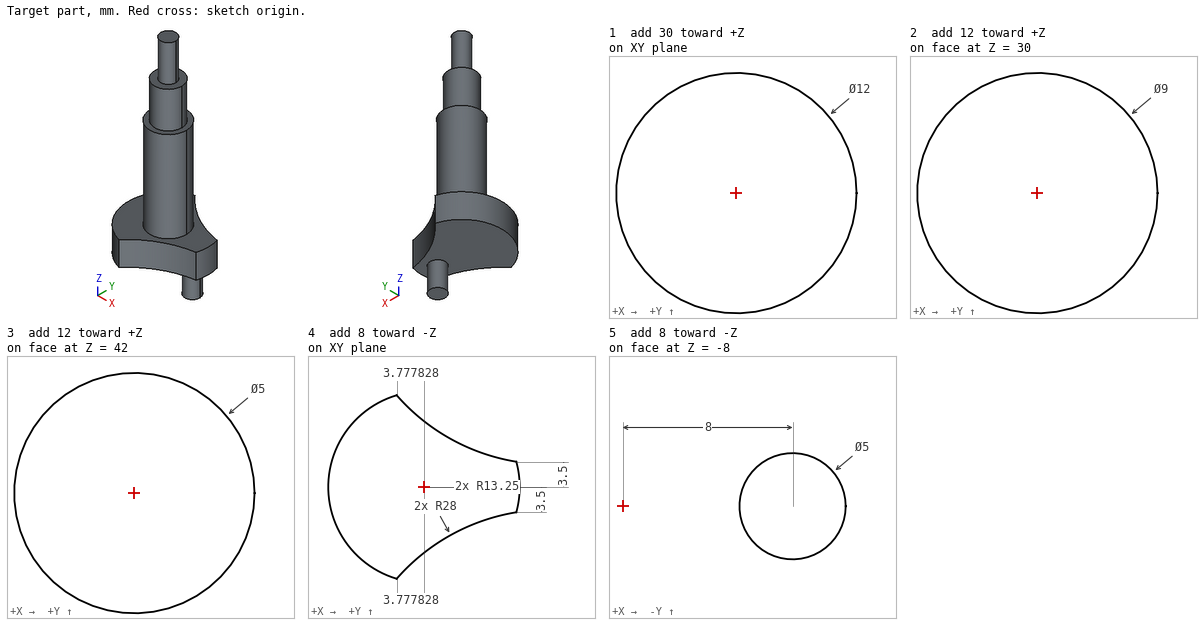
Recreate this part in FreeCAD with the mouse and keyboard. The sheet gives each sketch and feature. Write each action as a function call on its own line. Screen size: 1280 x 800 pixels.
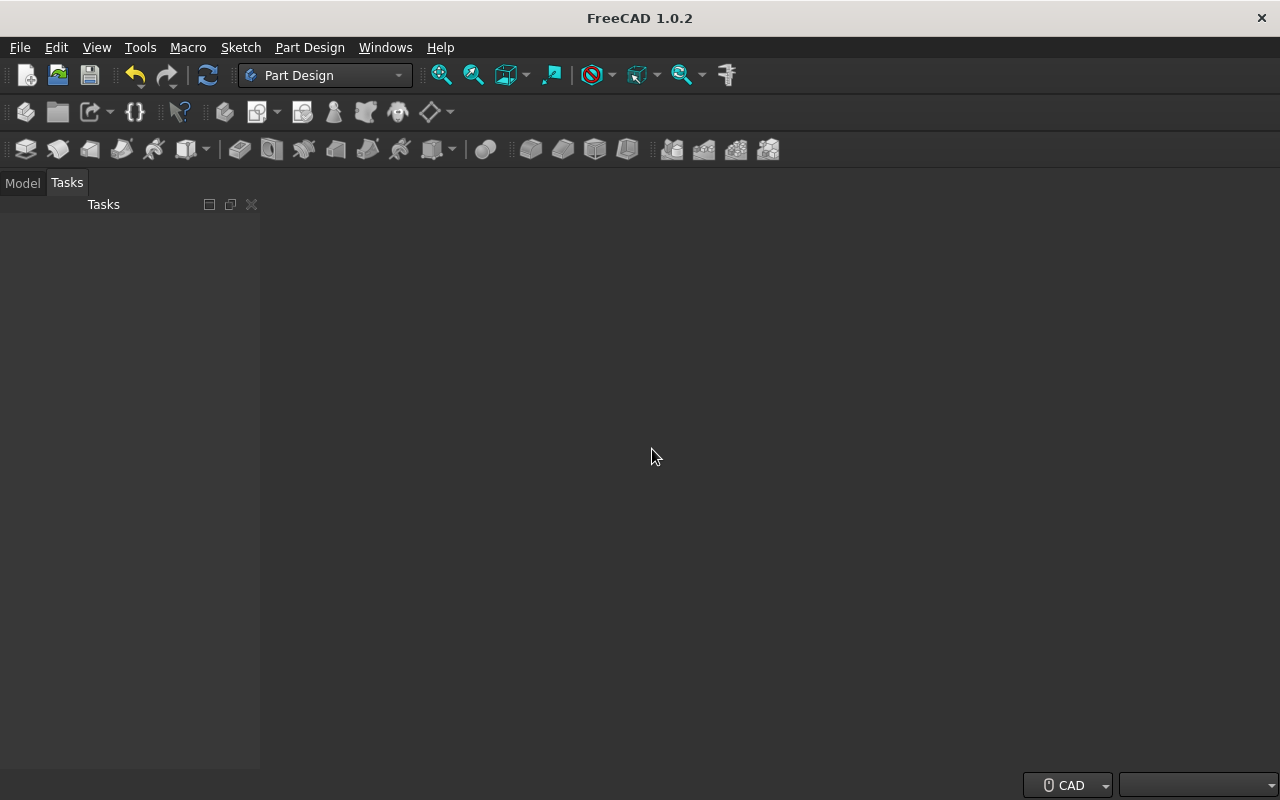
click(26, 76)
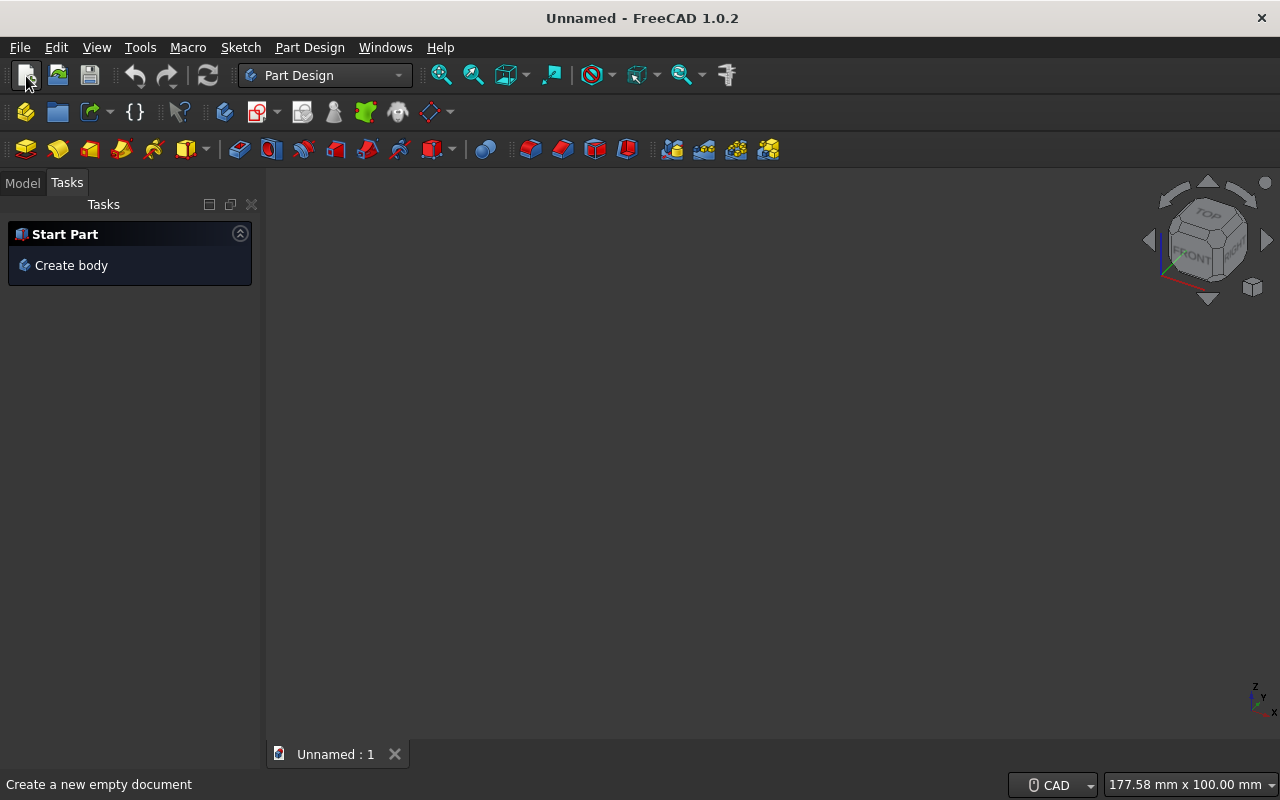
click(258, 112)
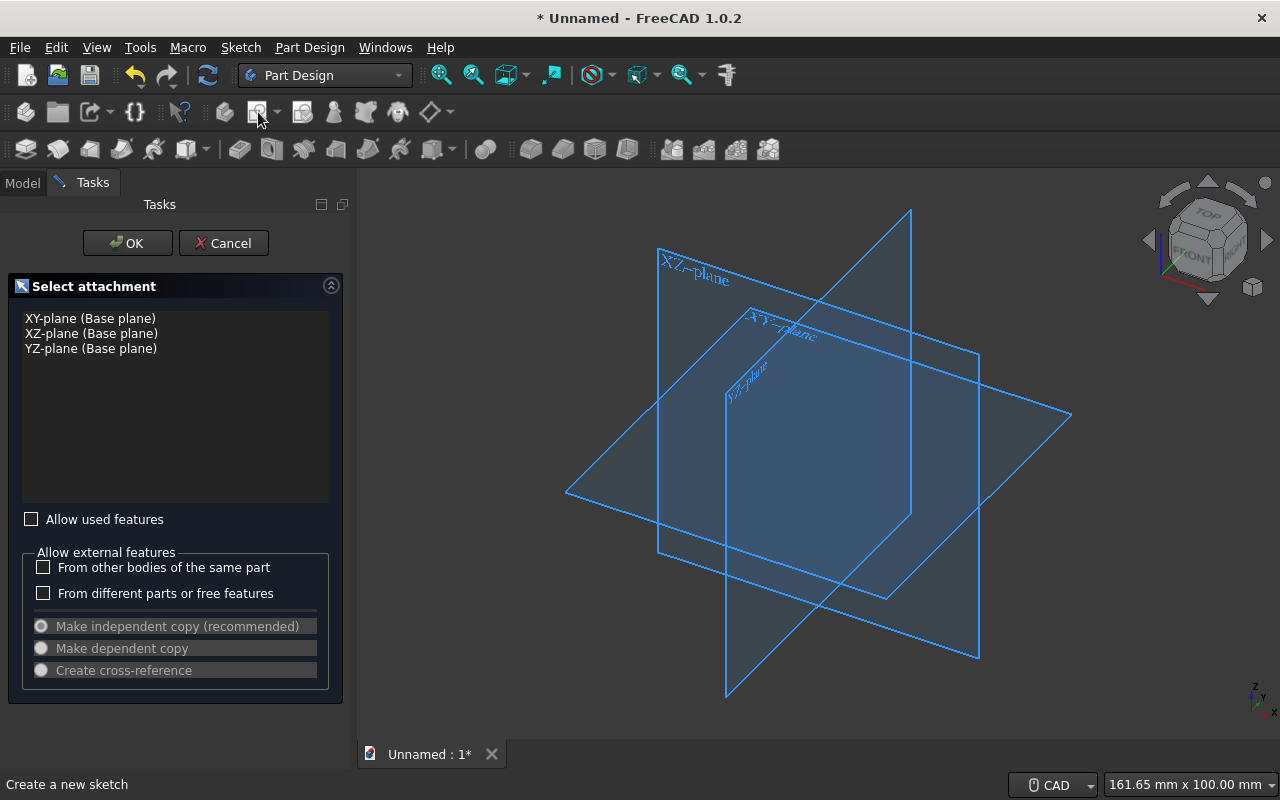
click(82, 318)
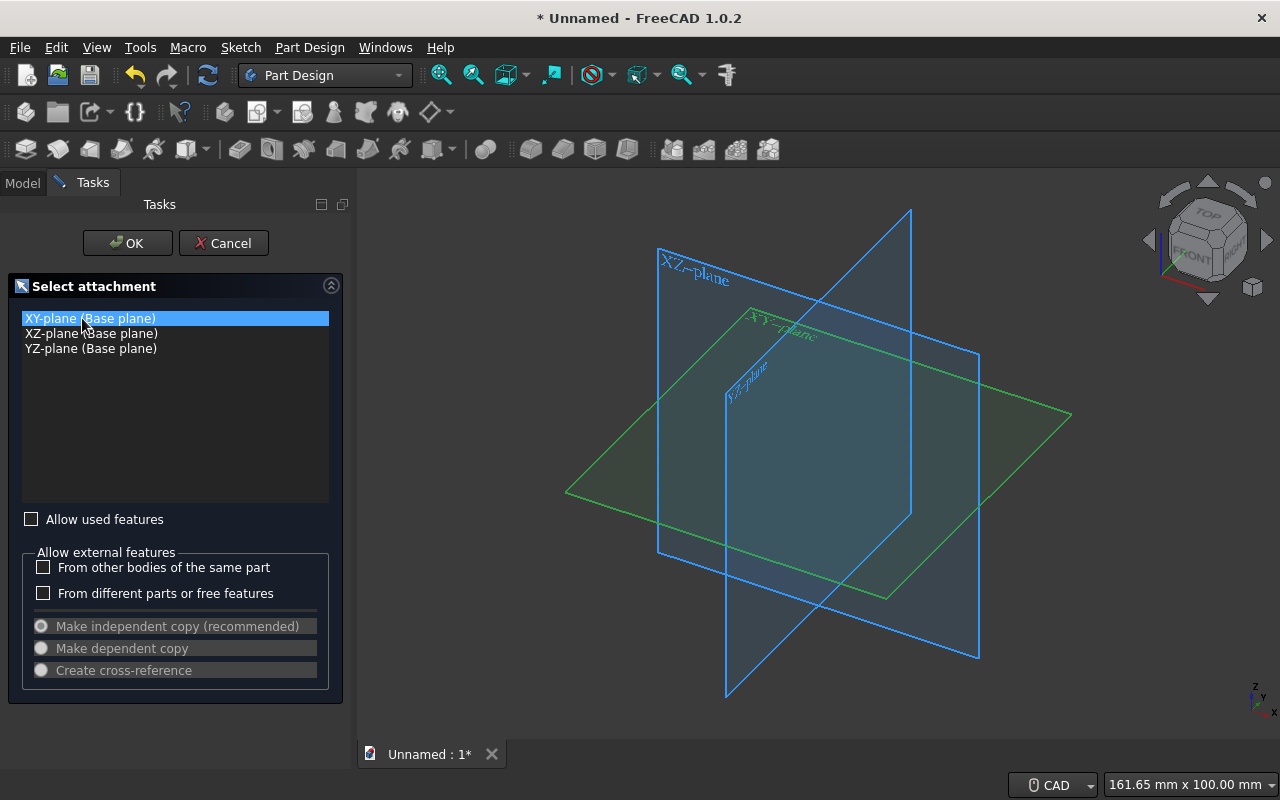
click(128, 243)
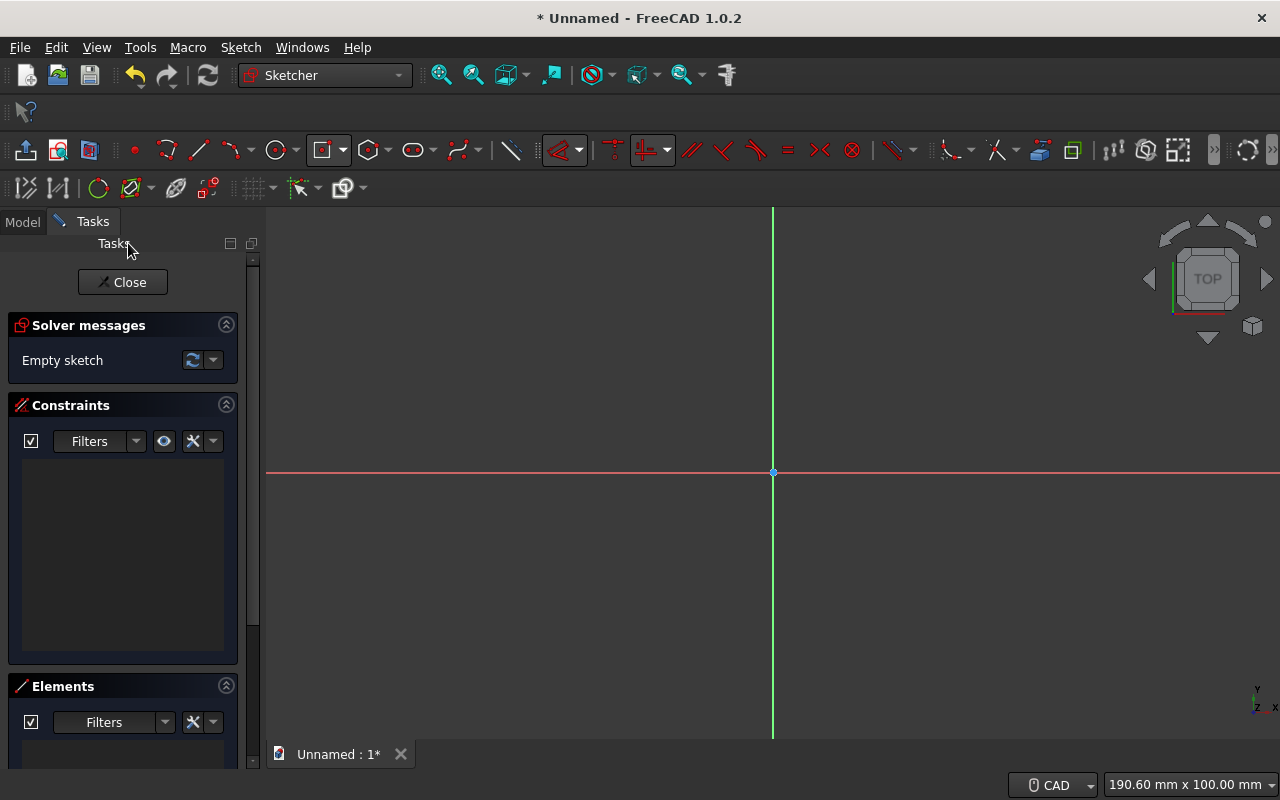
scroll(790, 473, up, 8)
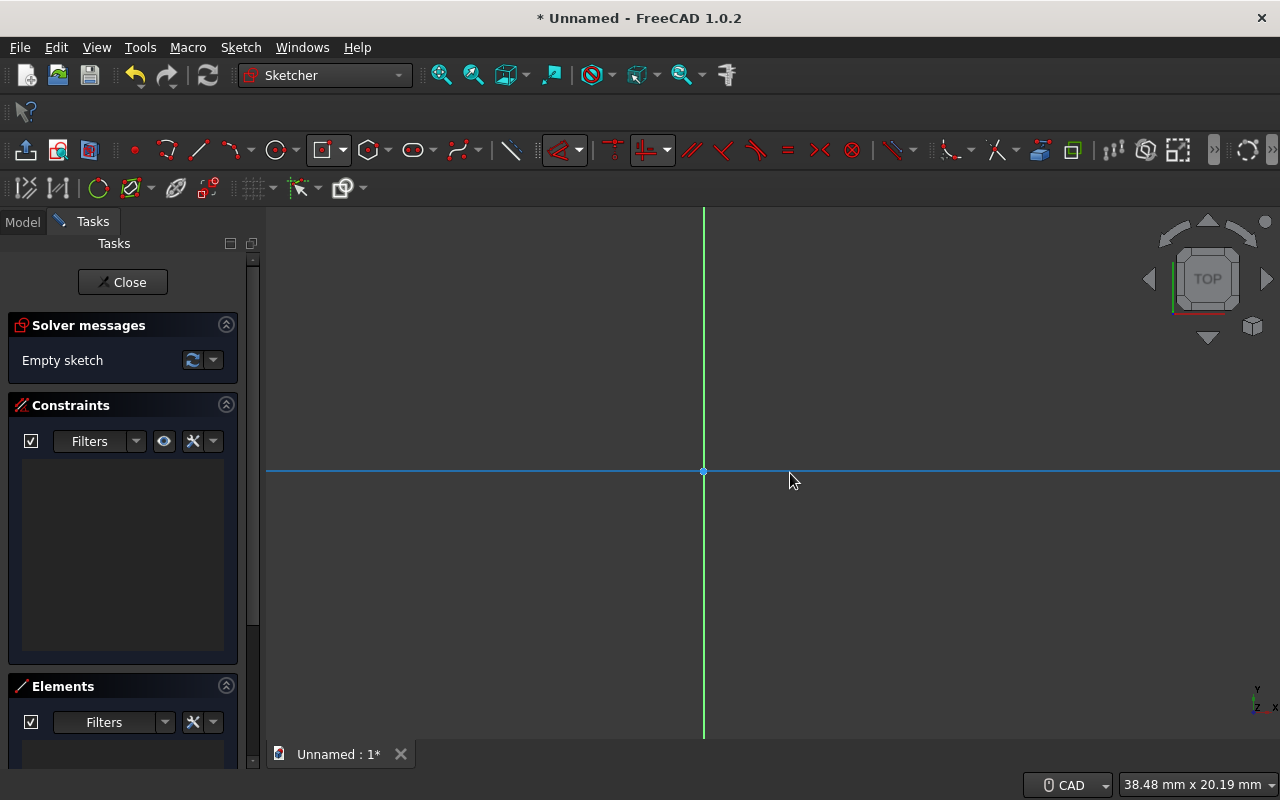
click(276, 150)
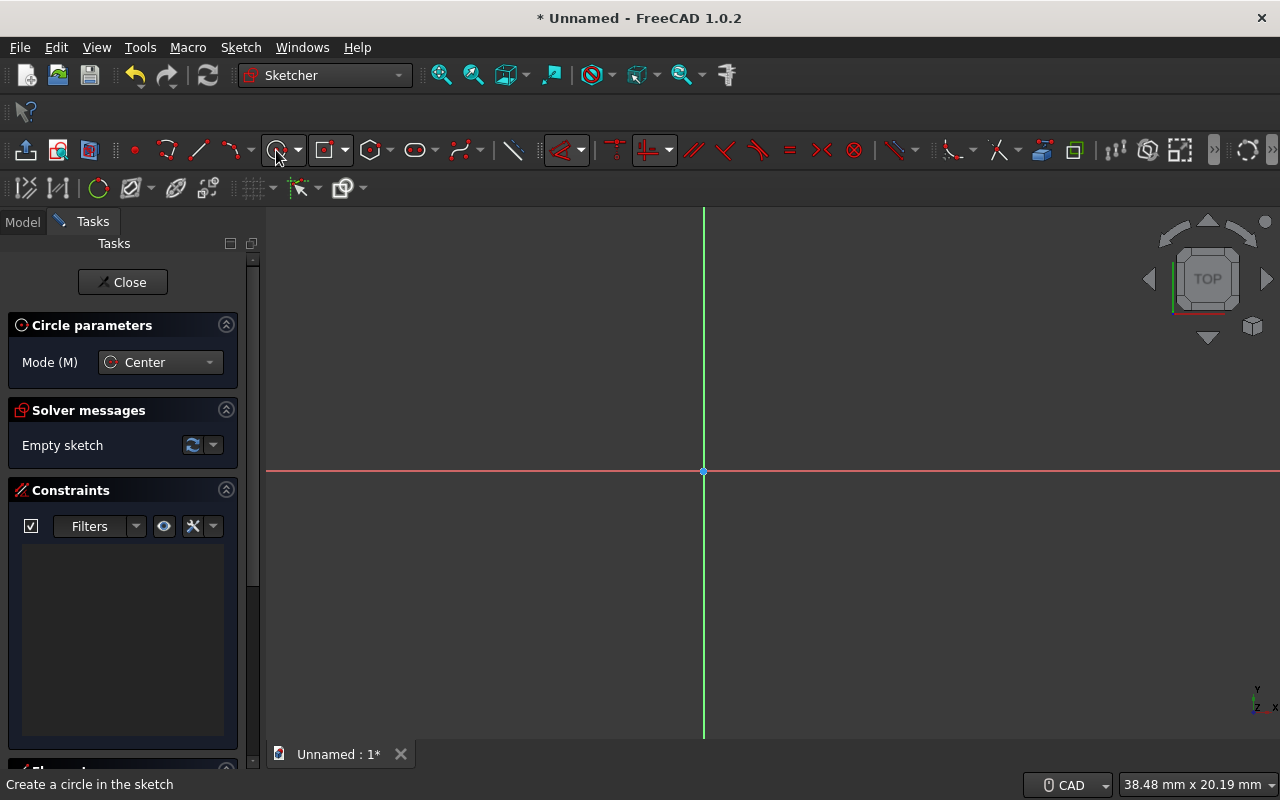
click(704, 471)
move(816, 359)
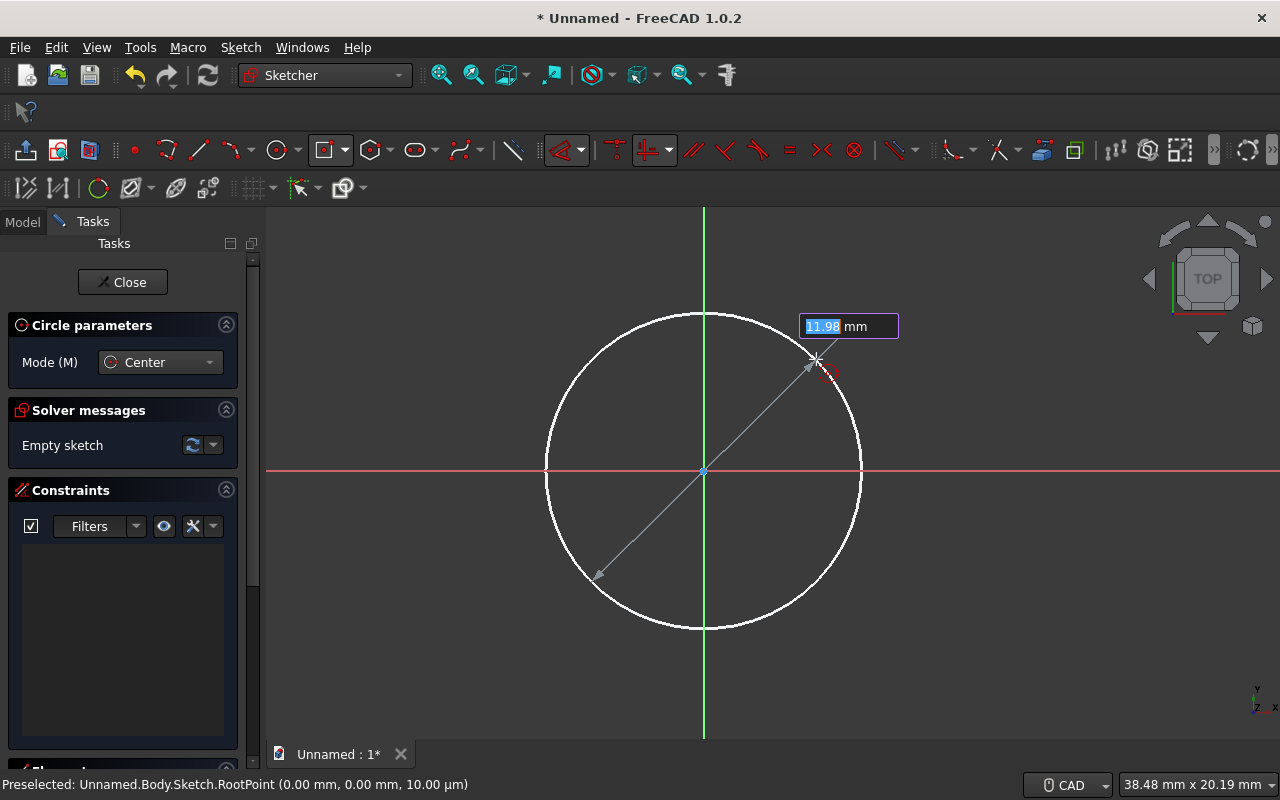
text(12)
key(Return)
key(Escape)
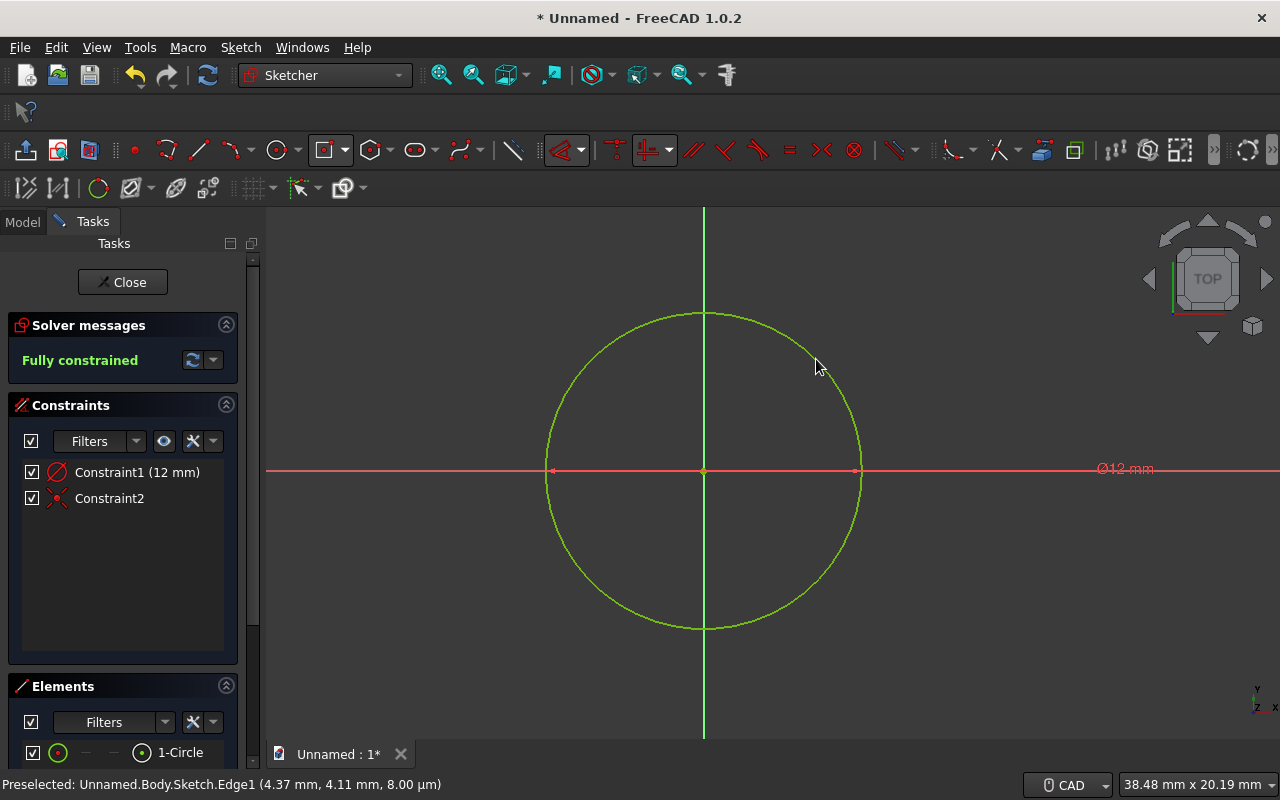
click(123, 282)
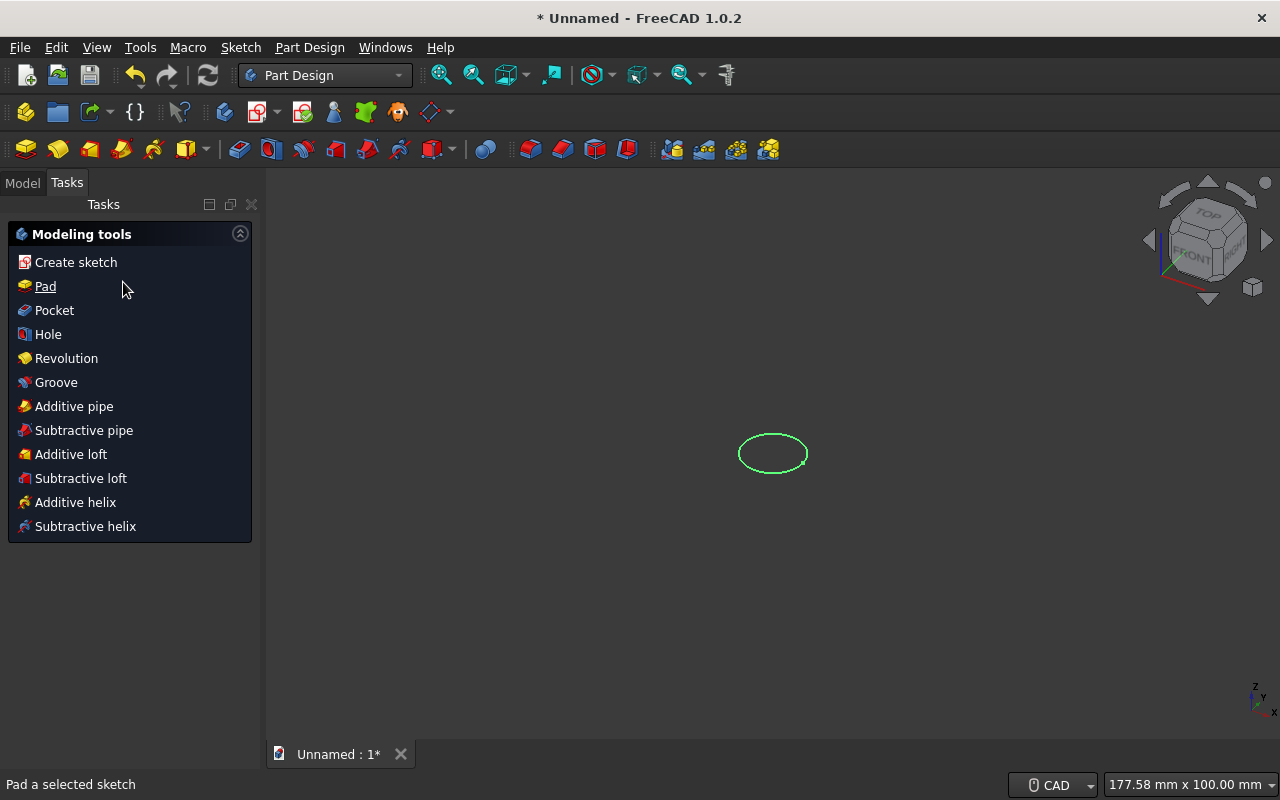
click(26, 150)